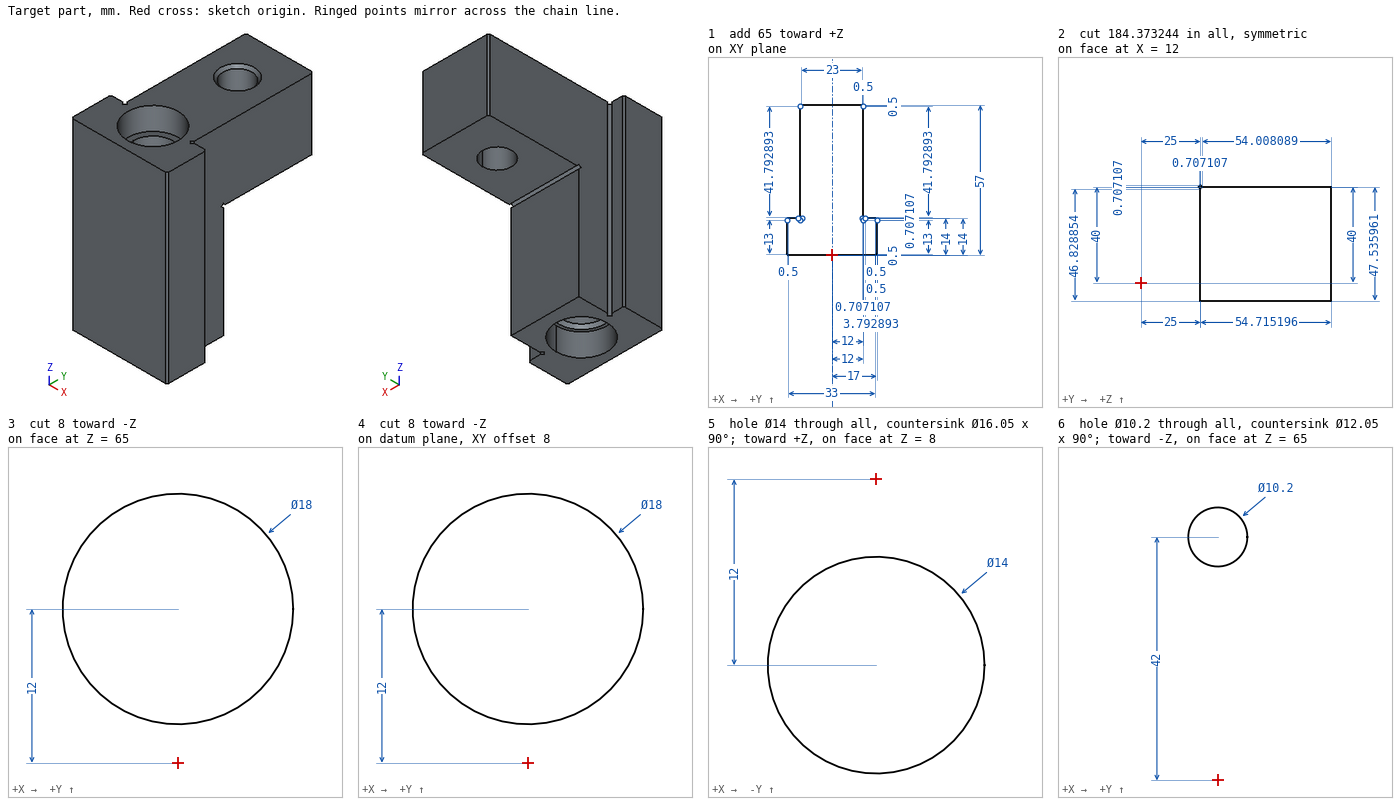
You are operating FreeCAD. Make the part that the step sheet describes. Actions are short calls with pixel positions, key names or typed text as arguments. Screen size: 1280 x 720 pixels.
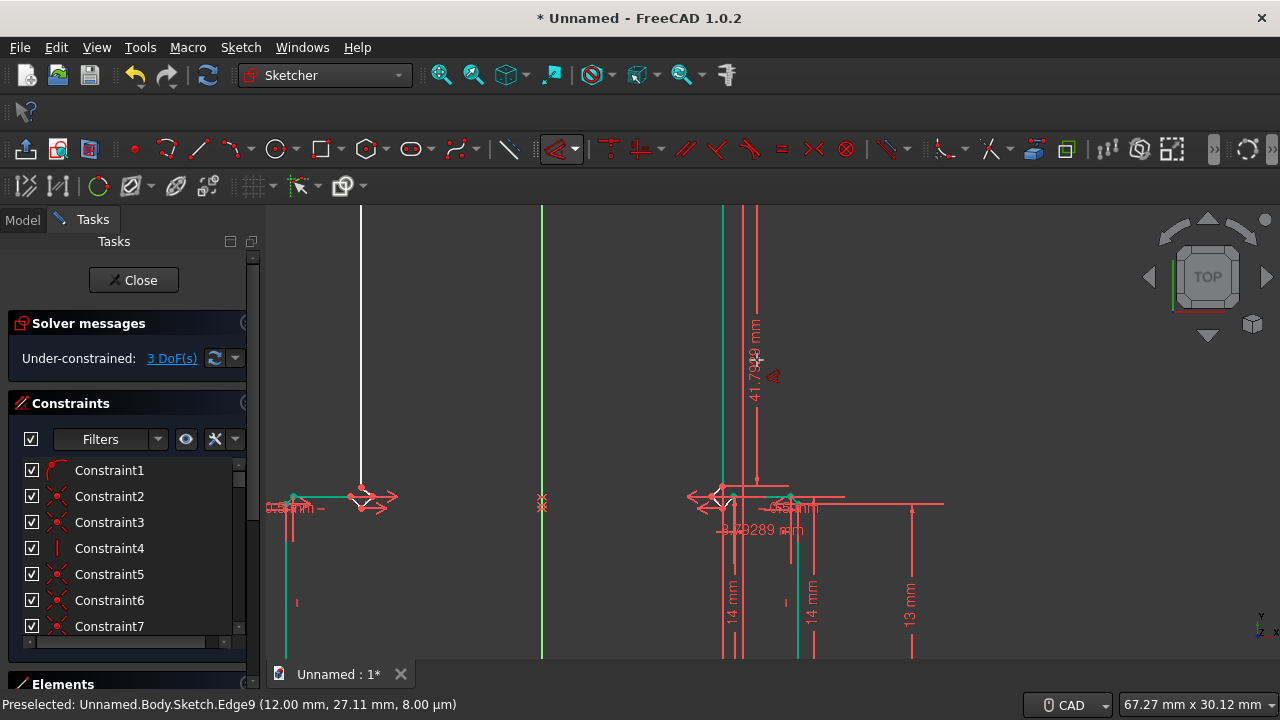
click(361, 298)
click(327, 360)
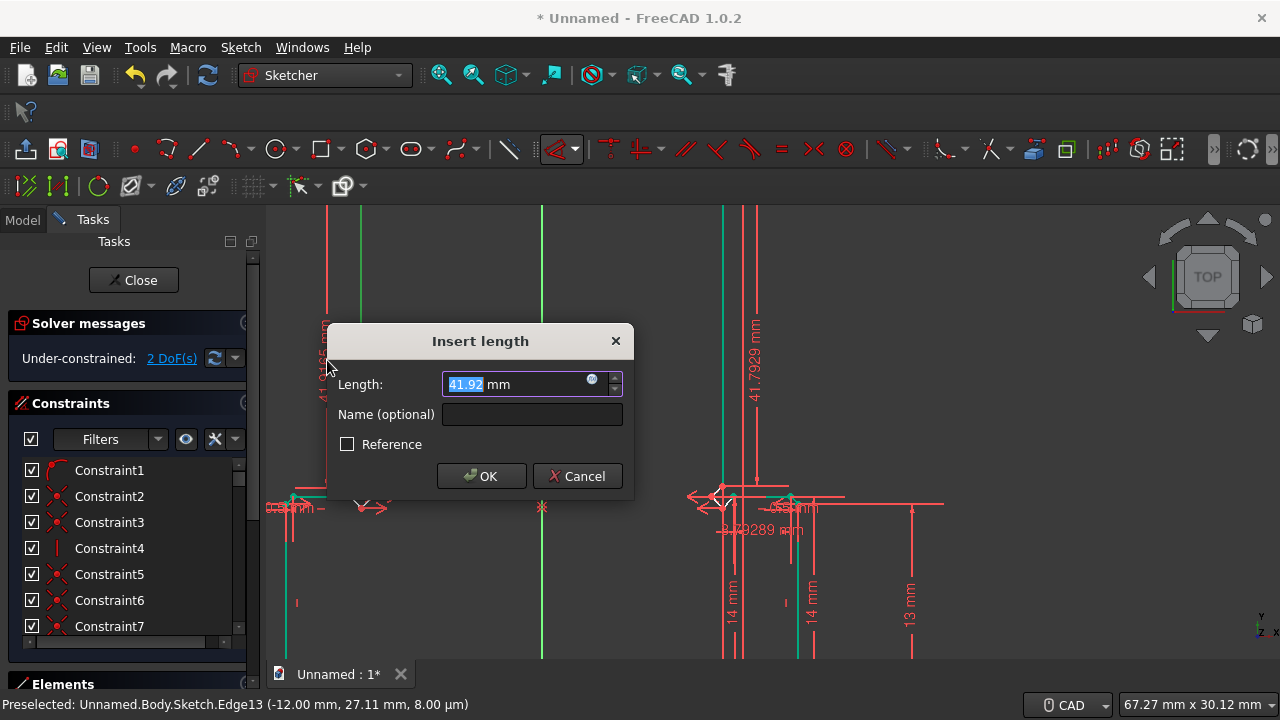
text(41.792893)
key(Return)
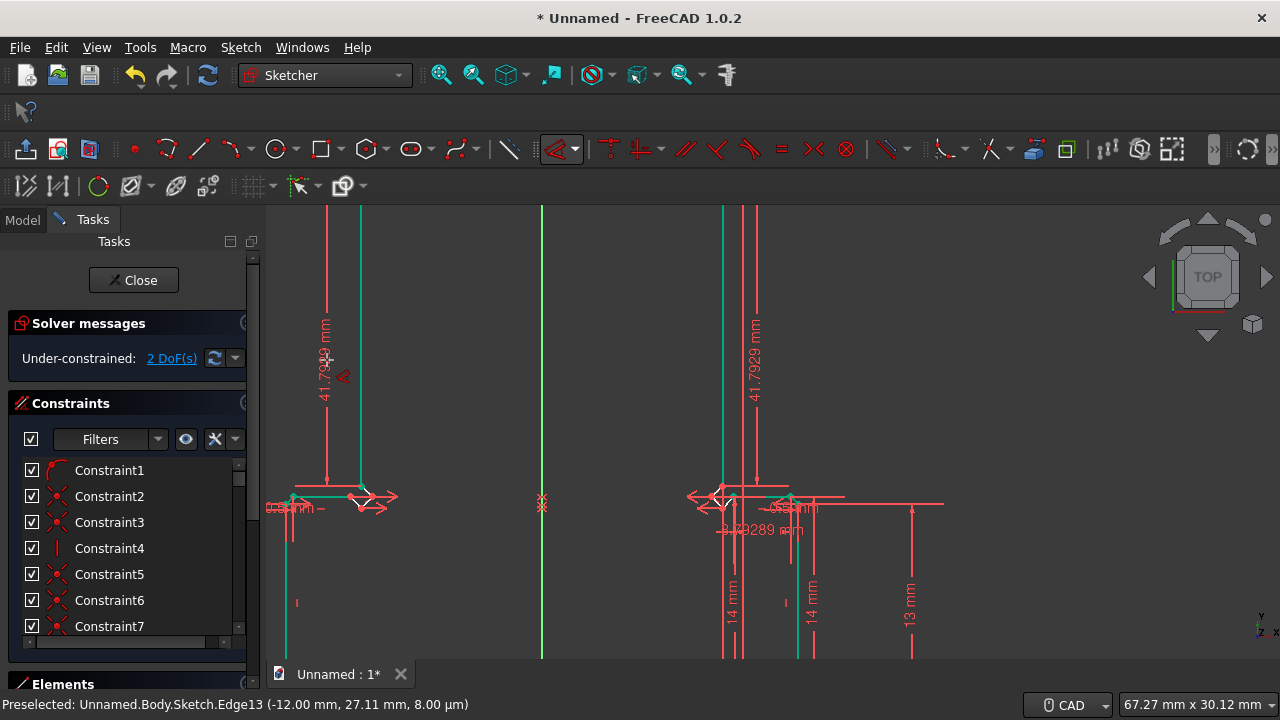
scroll(728, 503, up, 7)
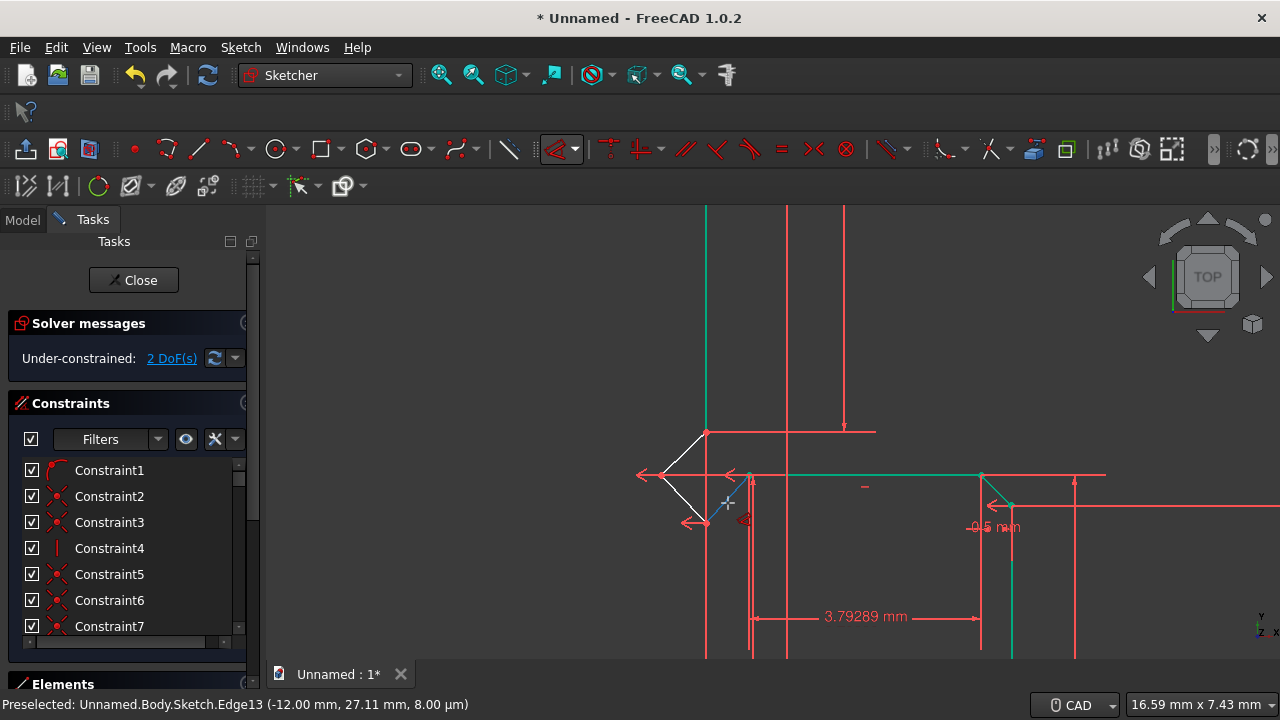
click(728, 499)
click(783, 499)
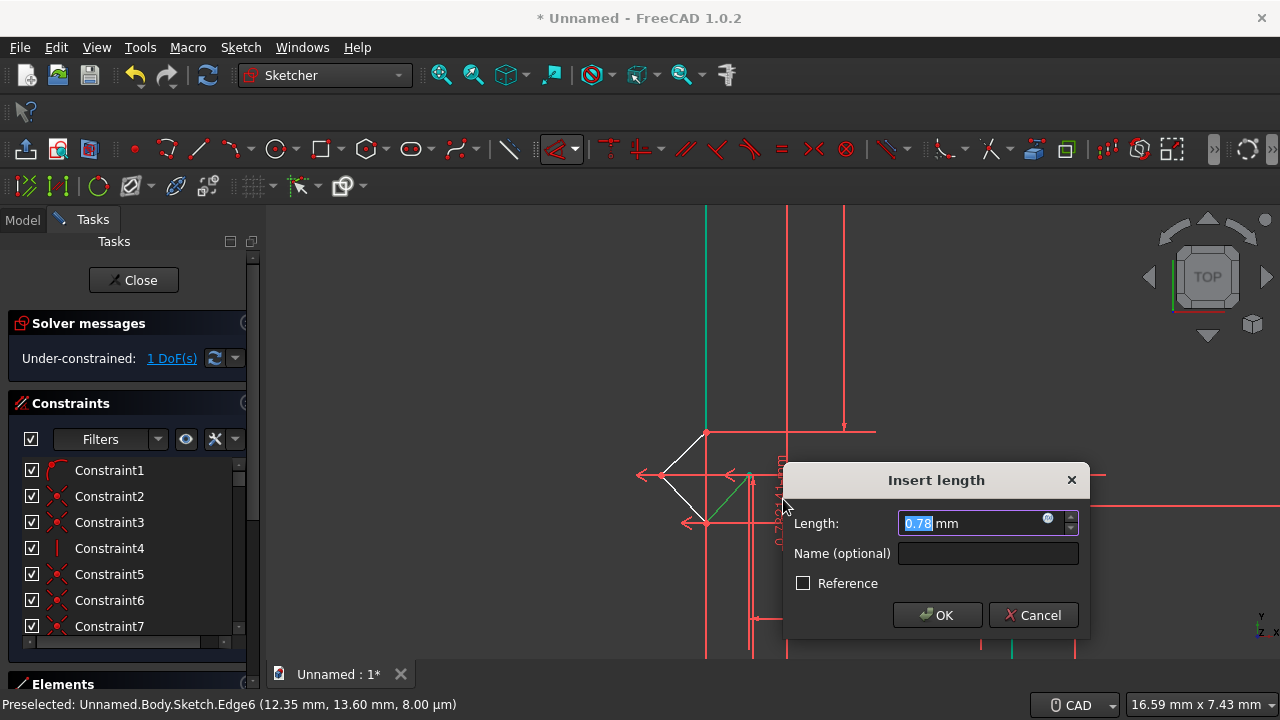
text(0.707107)
key(Return)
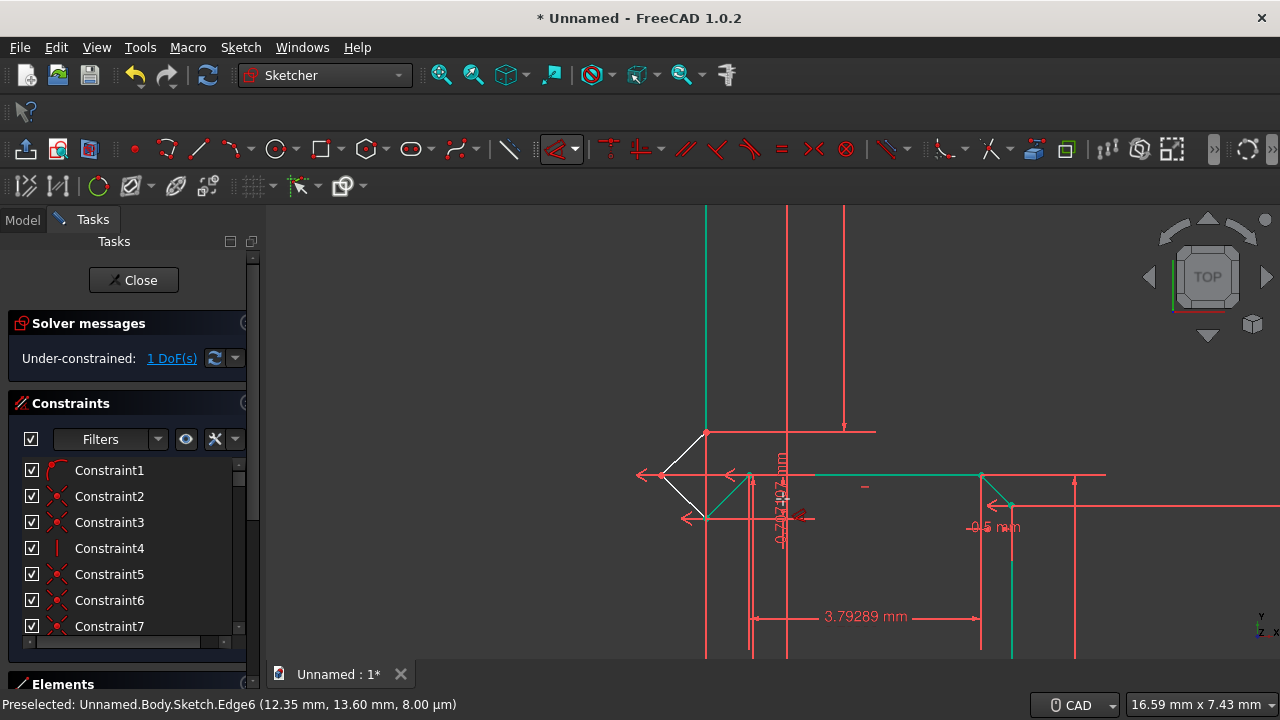
click(693, 506)
click(684, 553)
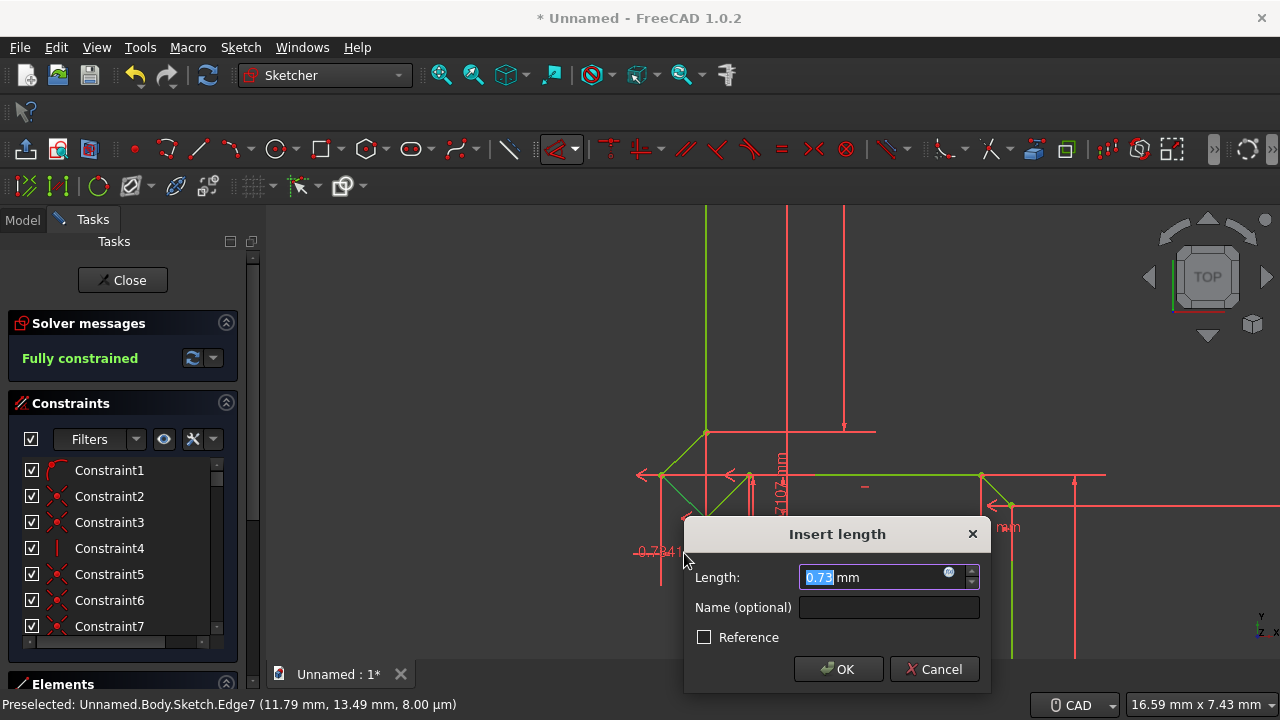
text(0.707107)
key(Return)
key(Escape)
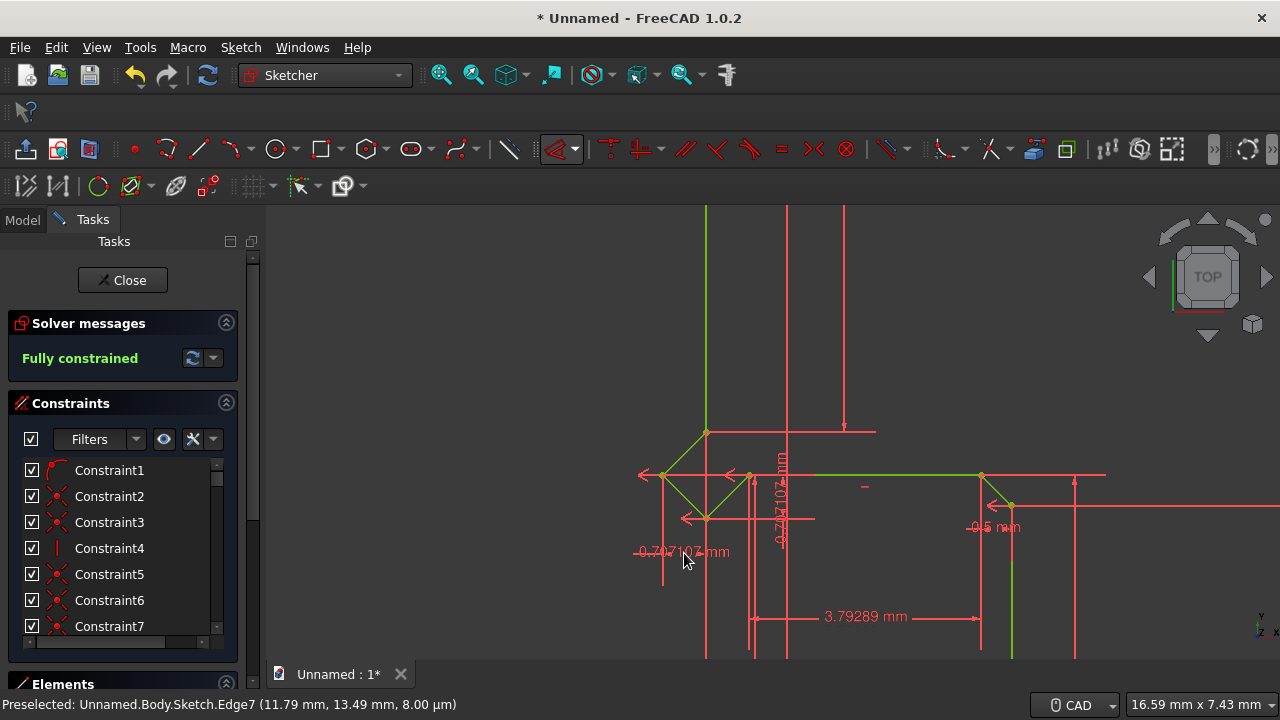
click(123, 280)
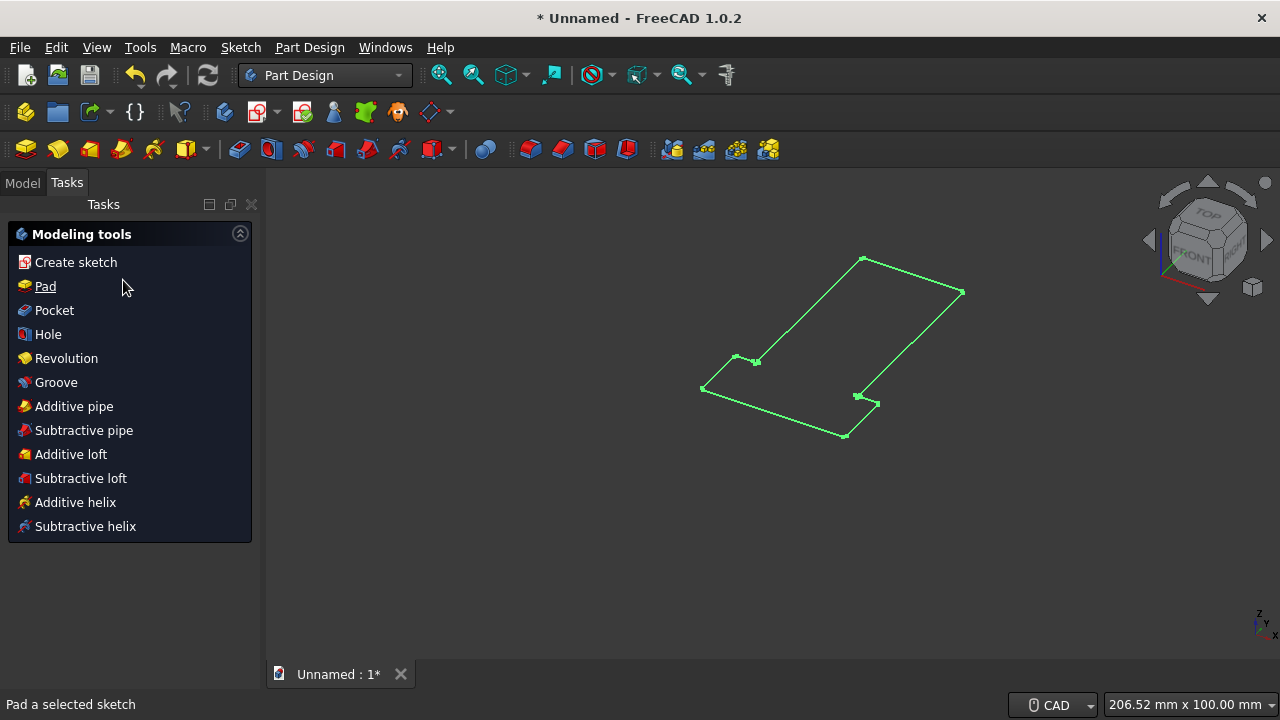
click(26, 150)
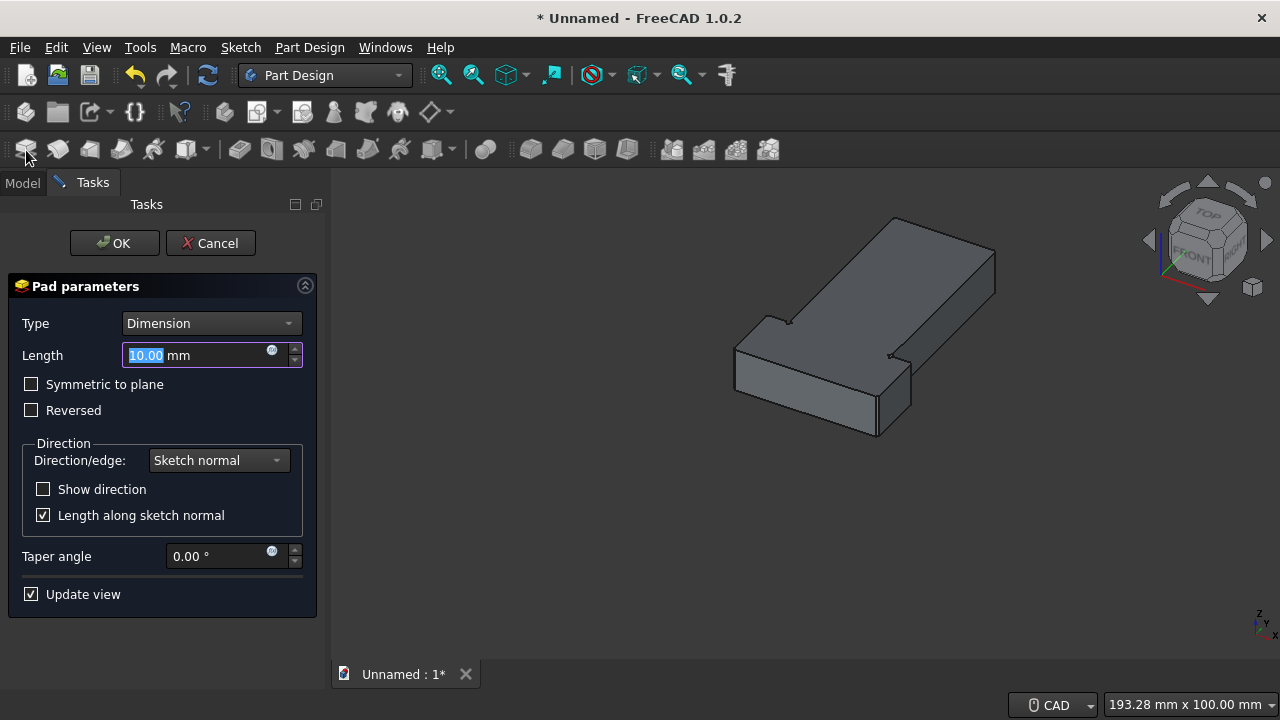
text(65)
key(Tab)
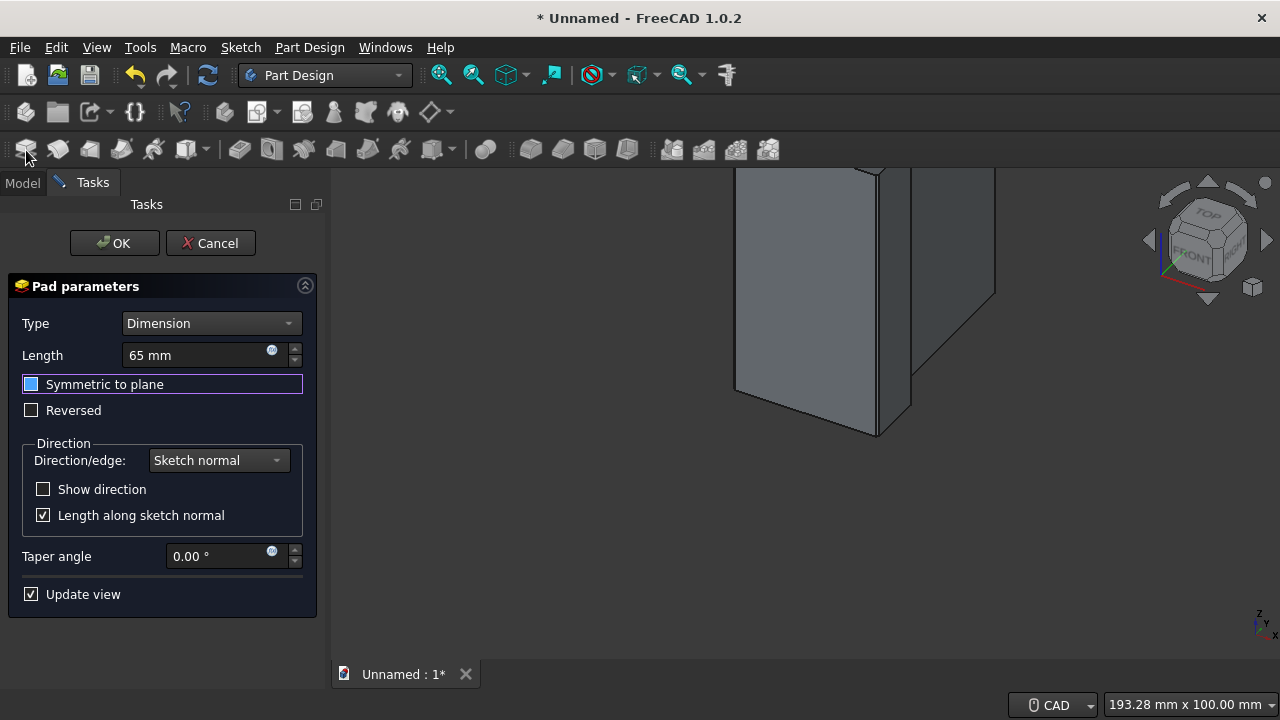
click(115, 243)